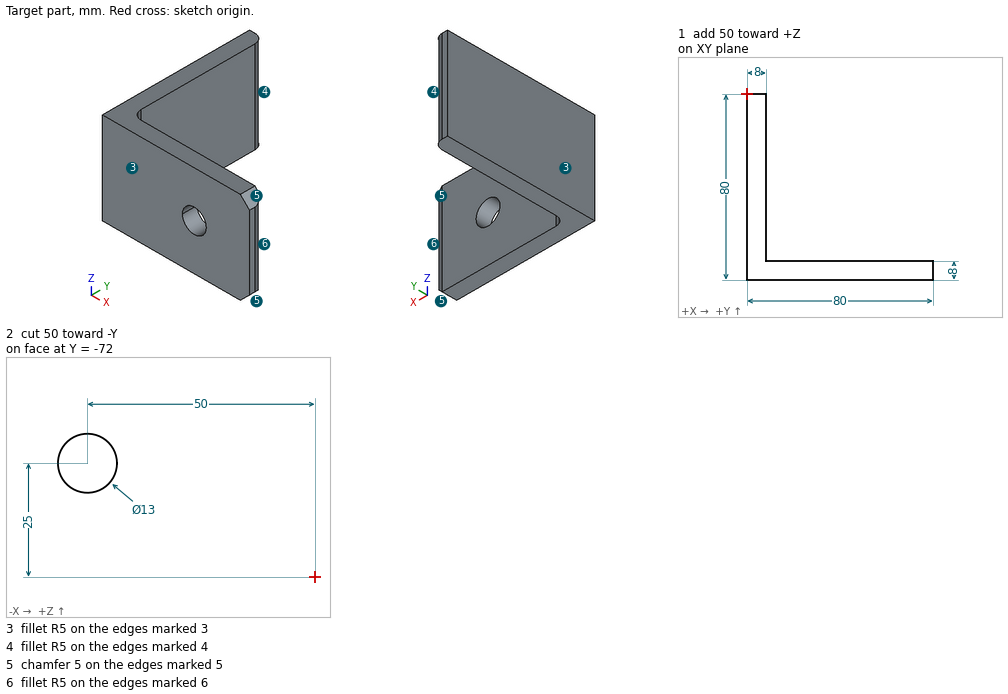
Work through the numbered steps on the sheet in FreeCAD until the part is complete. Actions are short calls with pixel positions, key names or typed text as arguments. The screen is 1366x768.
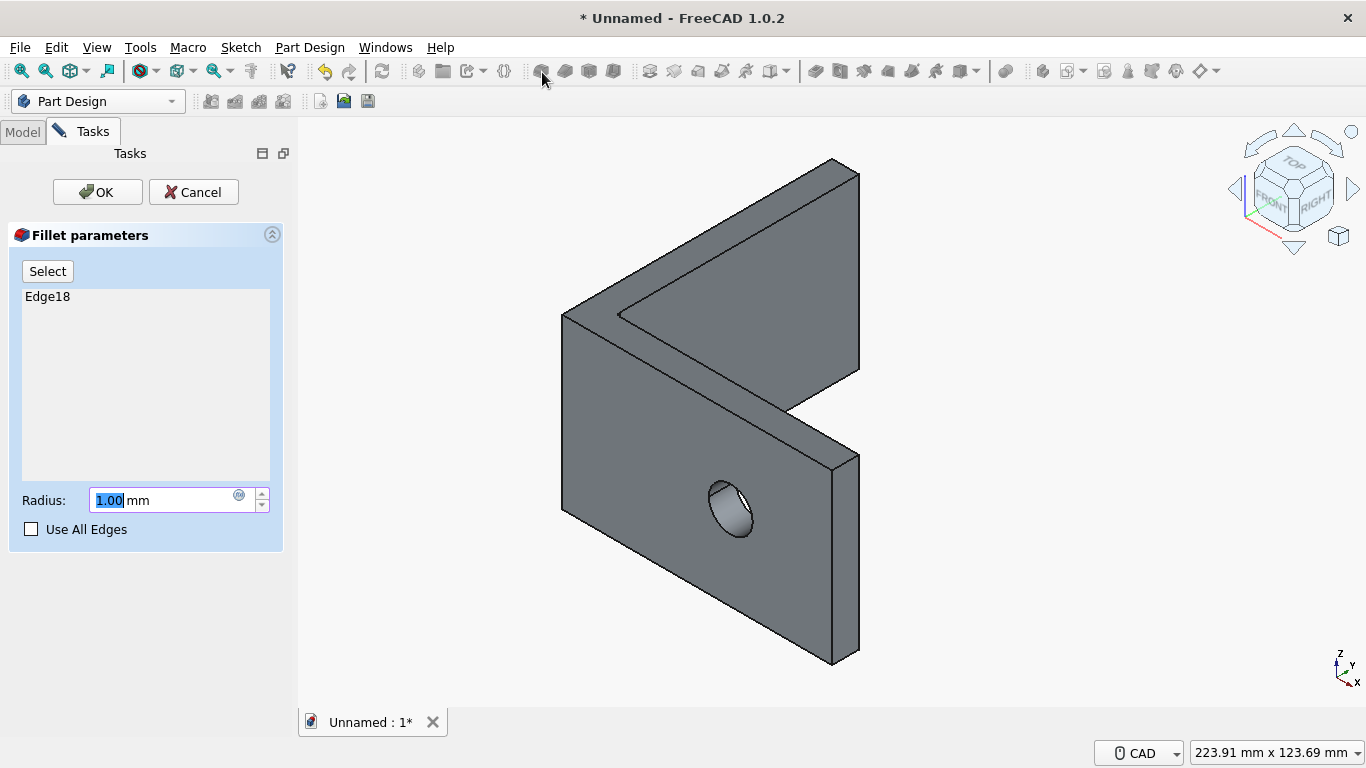
text(5)
key(Tab)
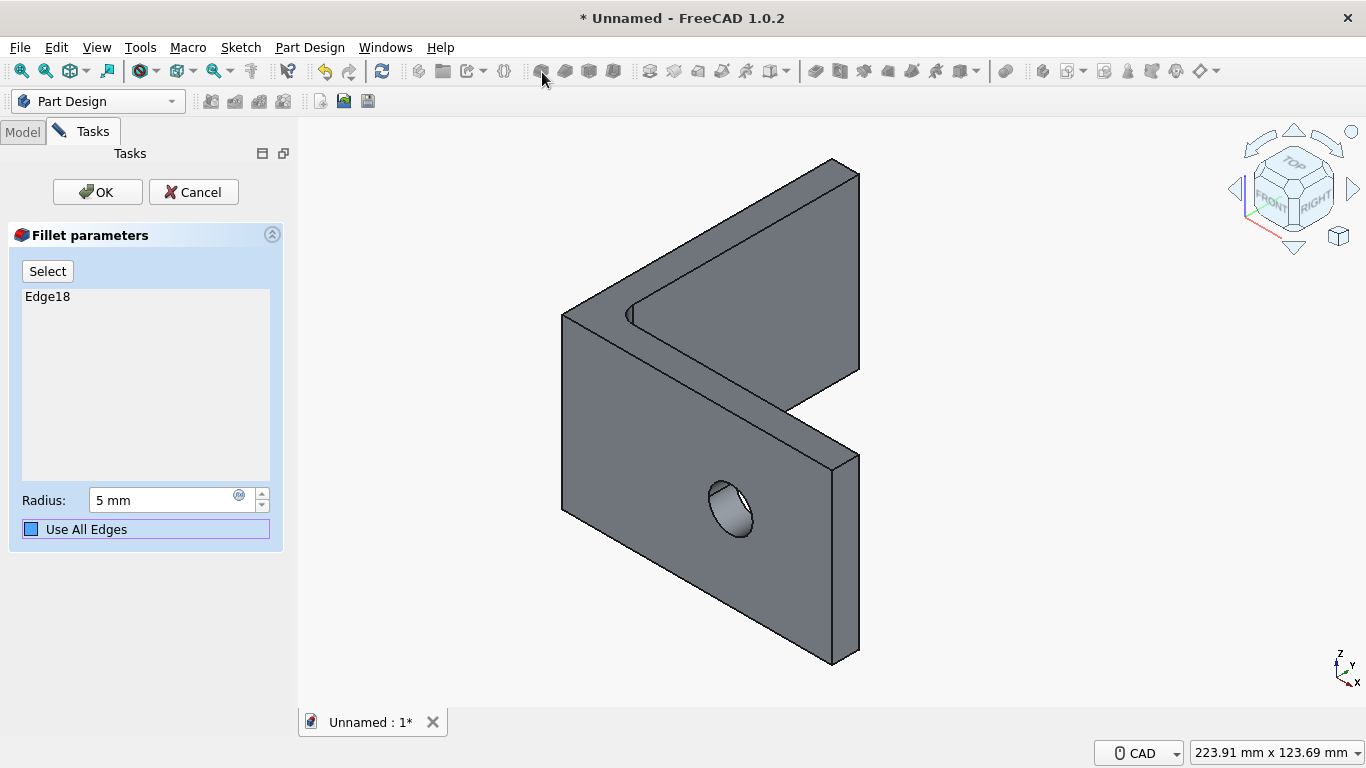
click(98, 192)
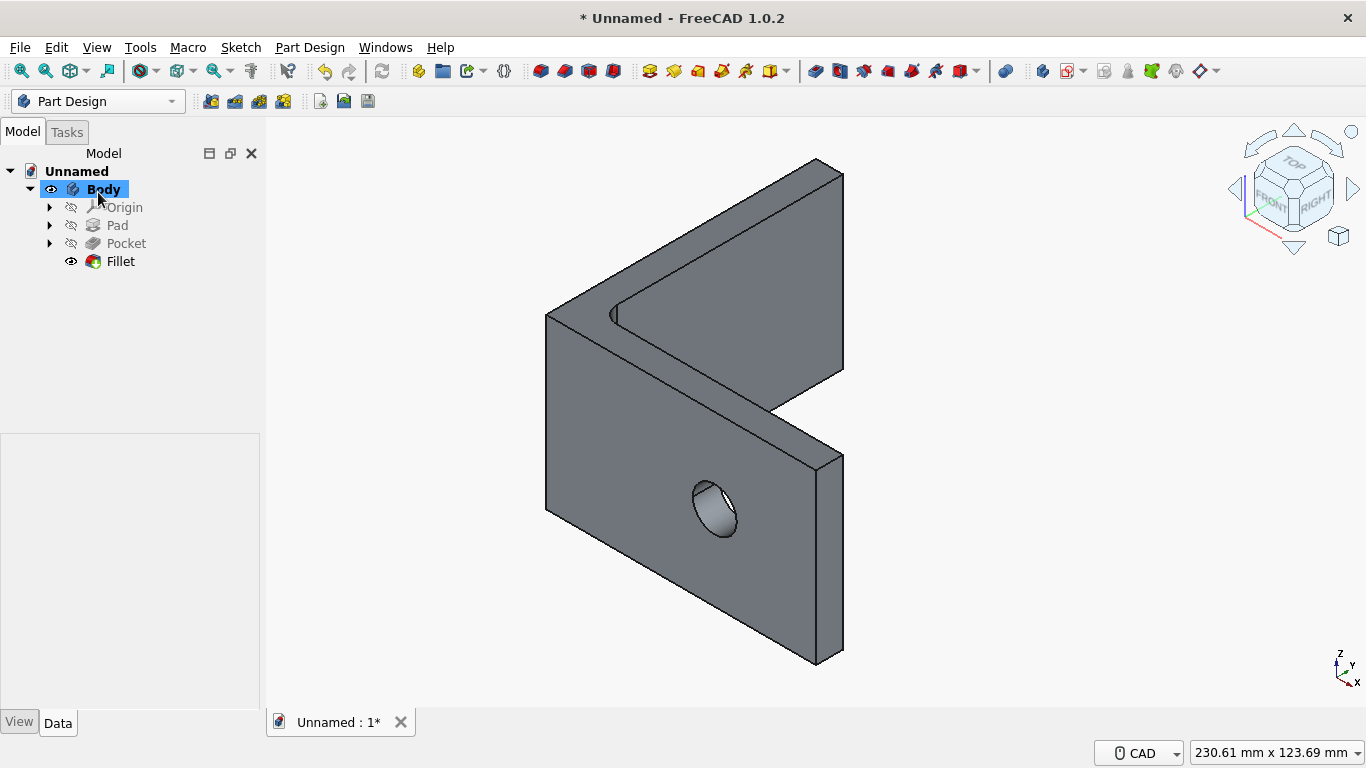
key(2)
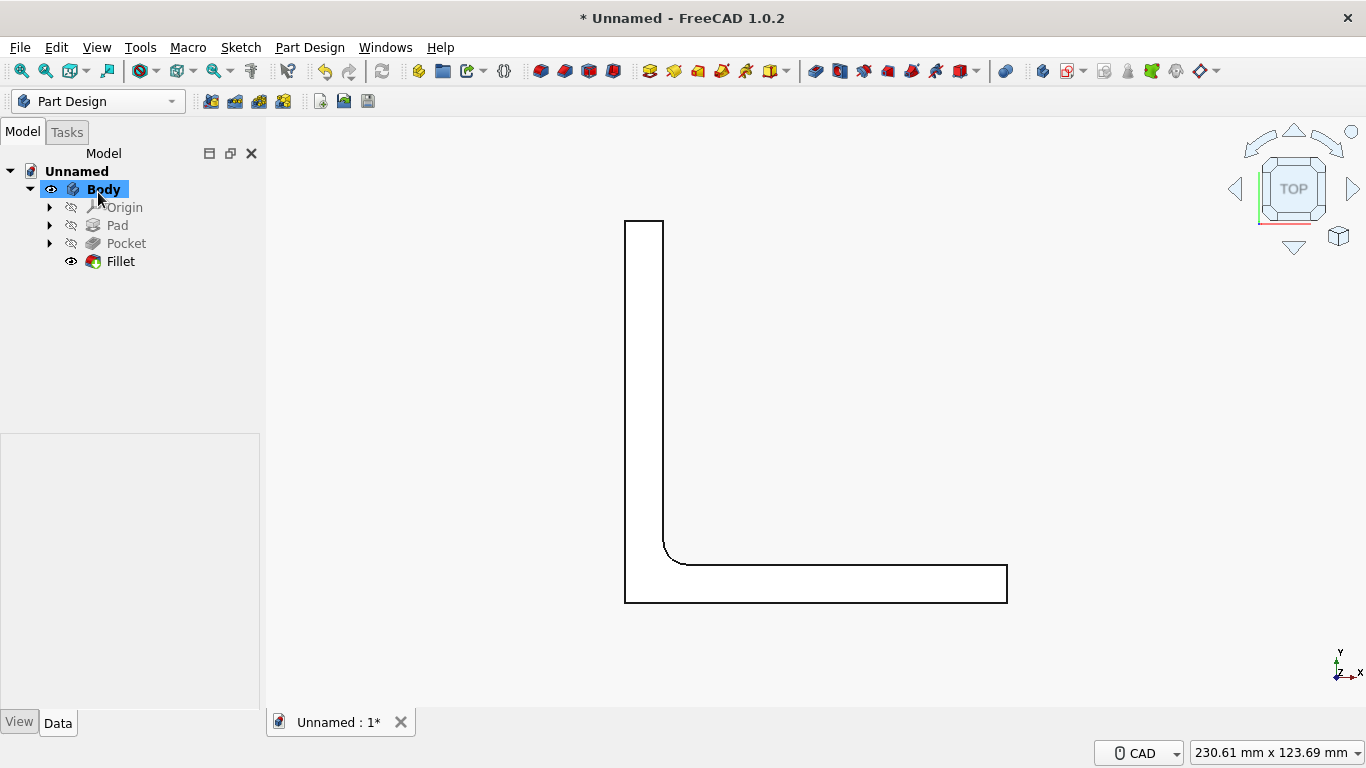
key(0)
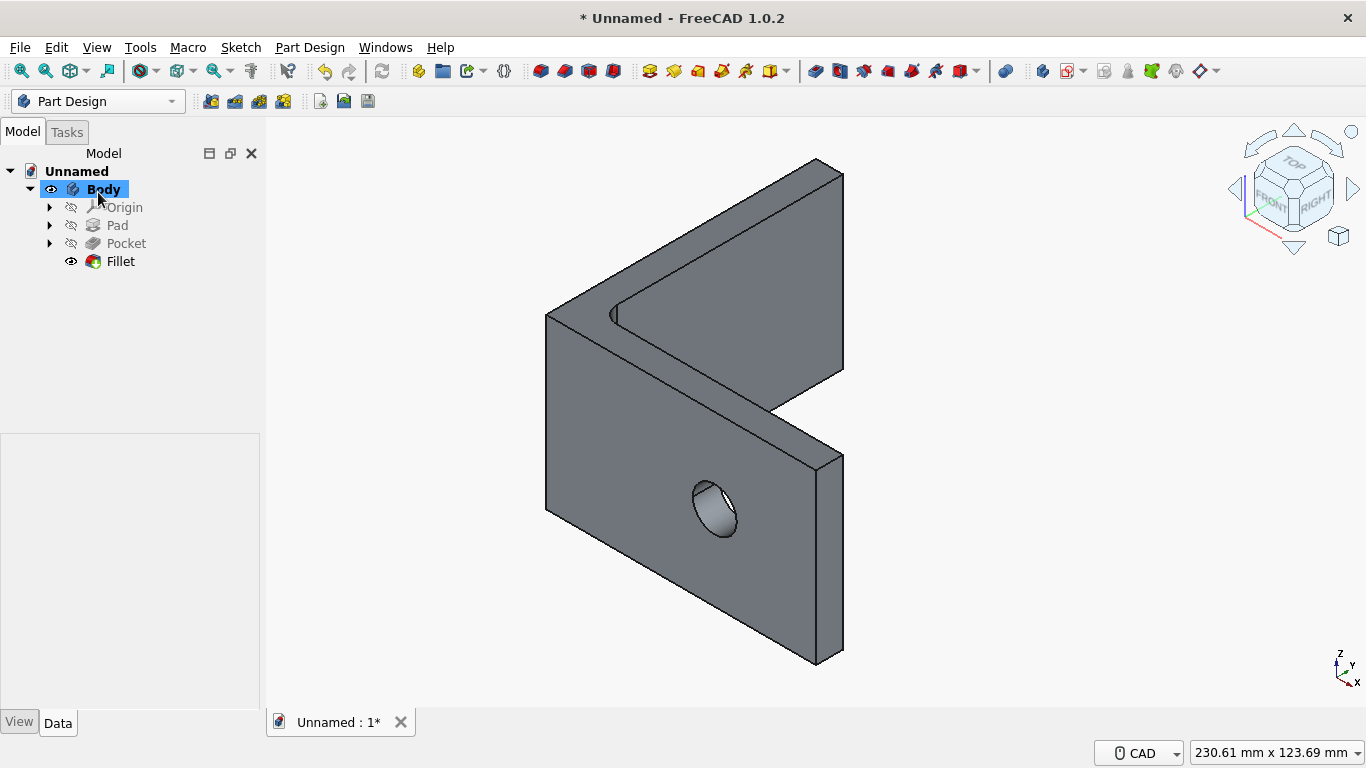
key(1)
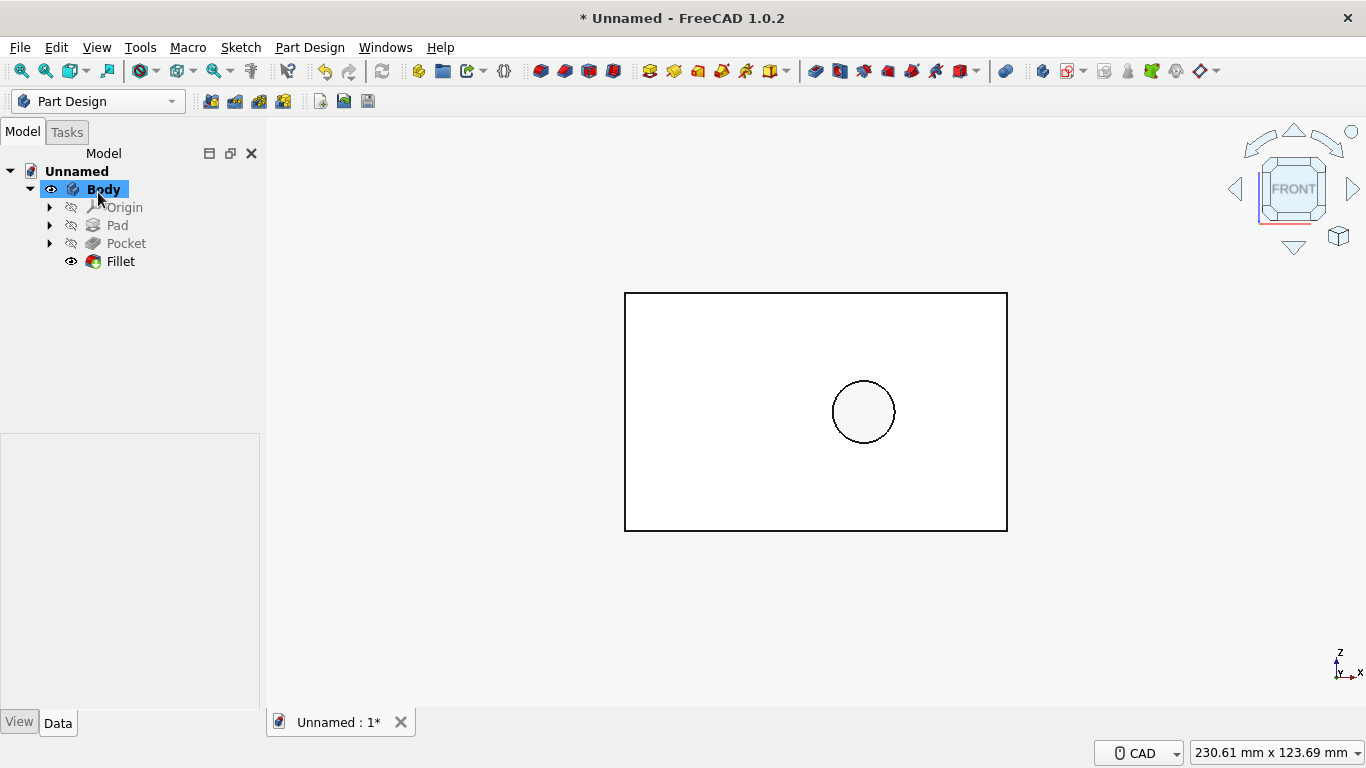
key(v)
key(f)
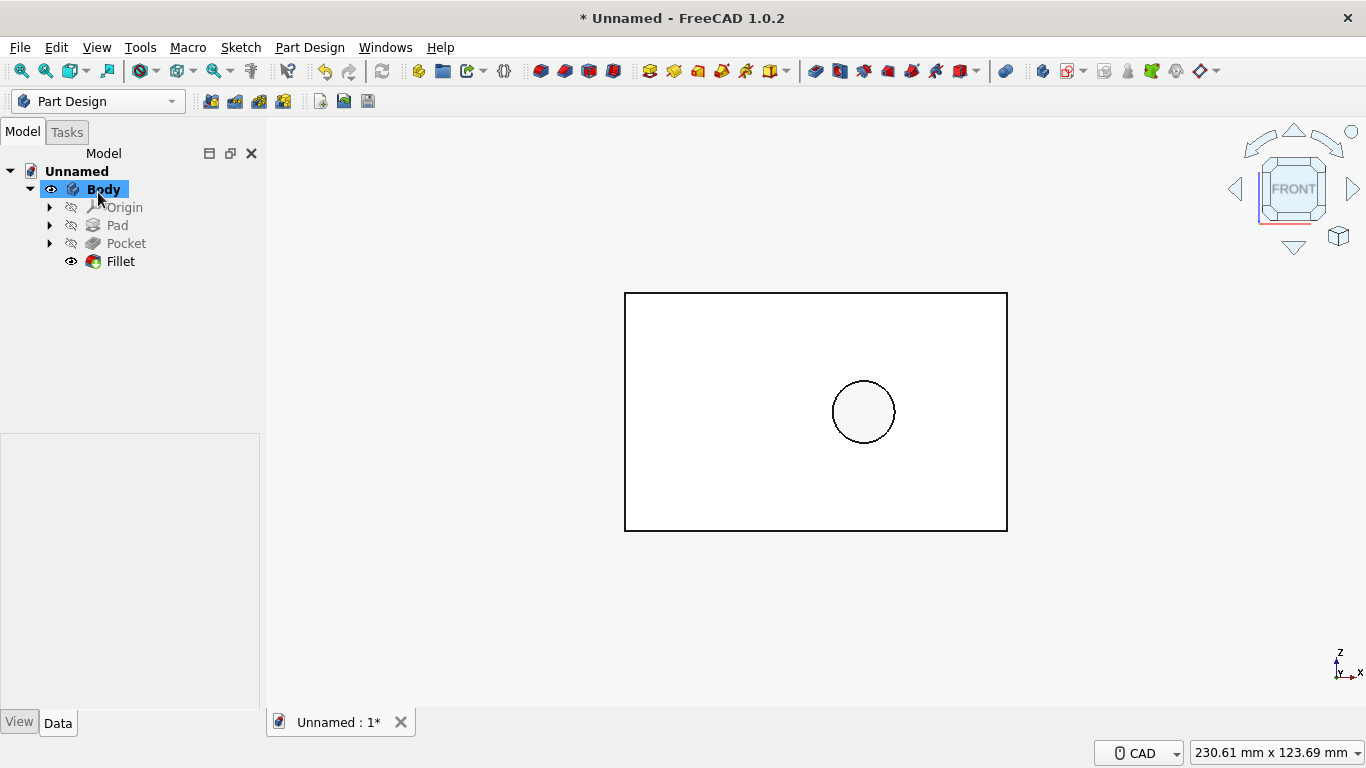
key(3)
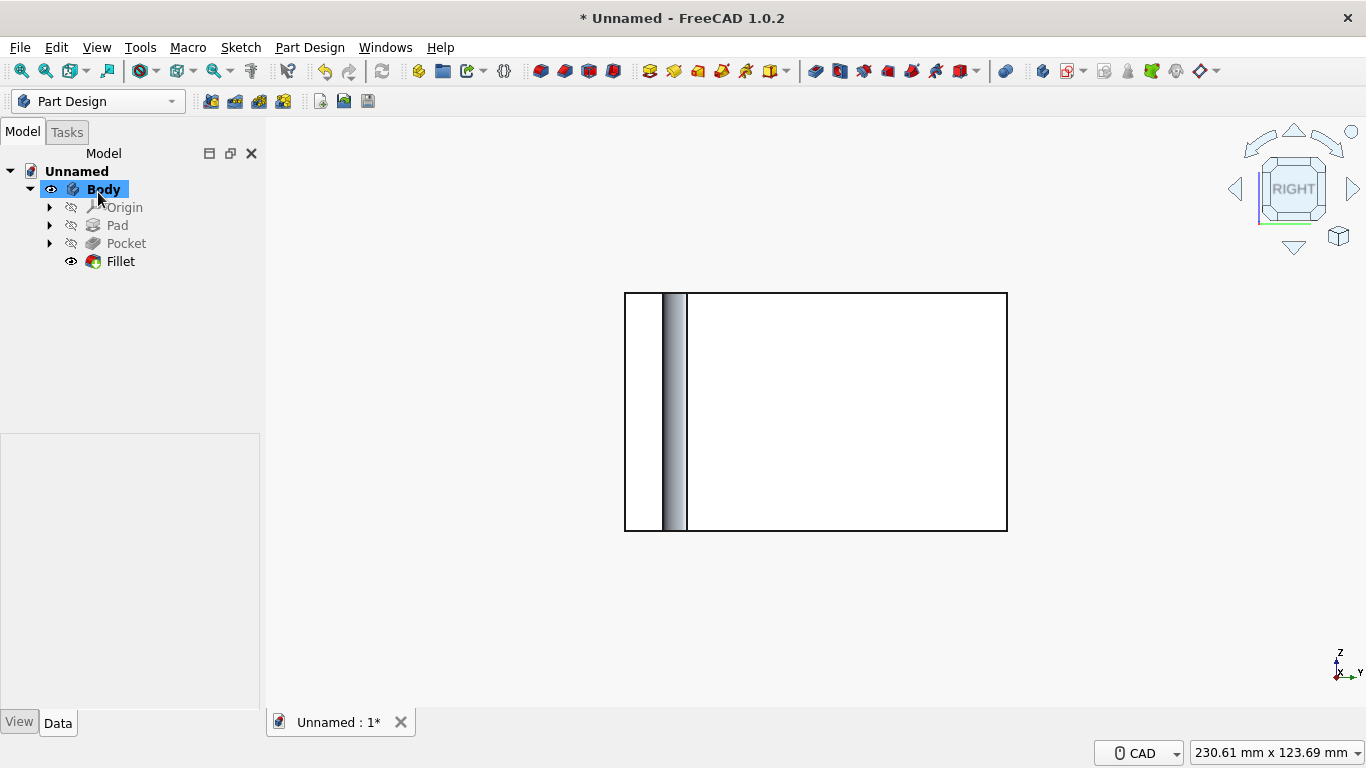
click(22, 72)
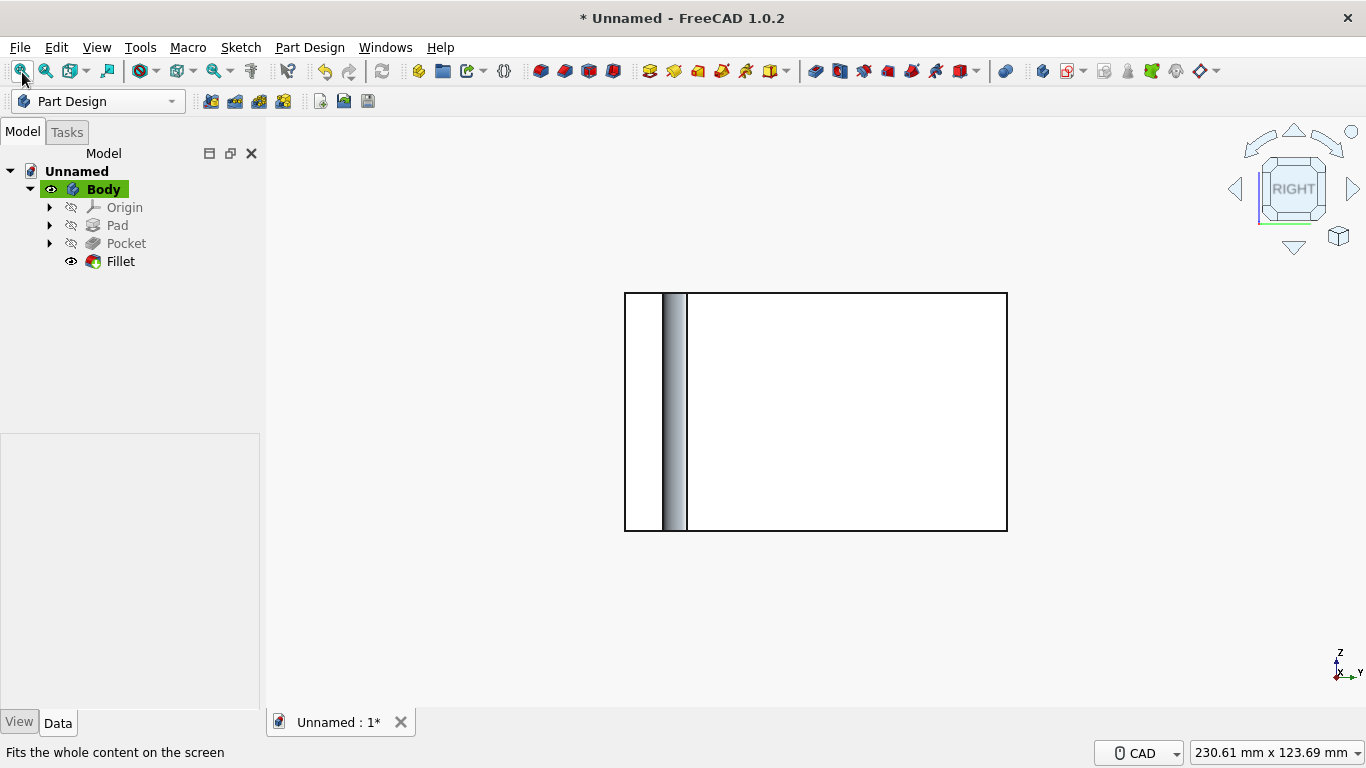
click(1007, 411)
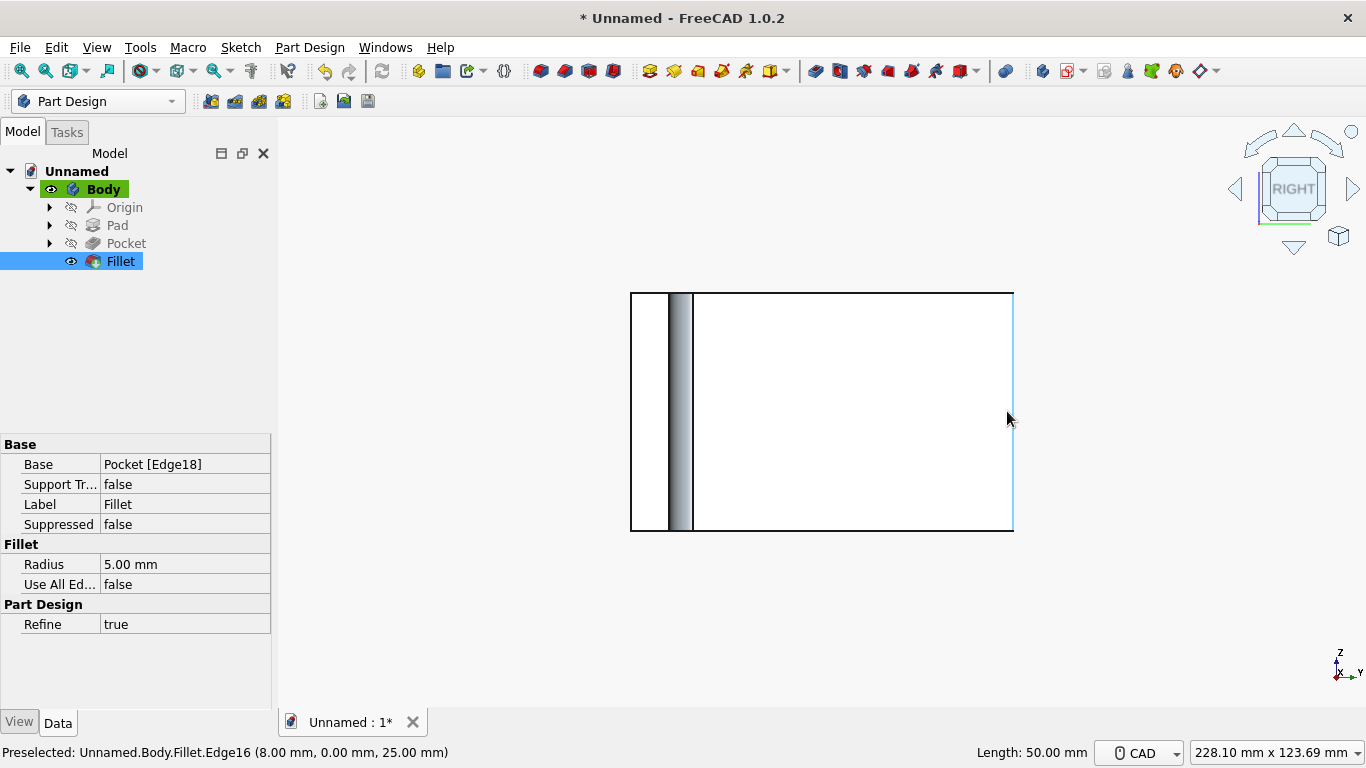
click(542, 72)